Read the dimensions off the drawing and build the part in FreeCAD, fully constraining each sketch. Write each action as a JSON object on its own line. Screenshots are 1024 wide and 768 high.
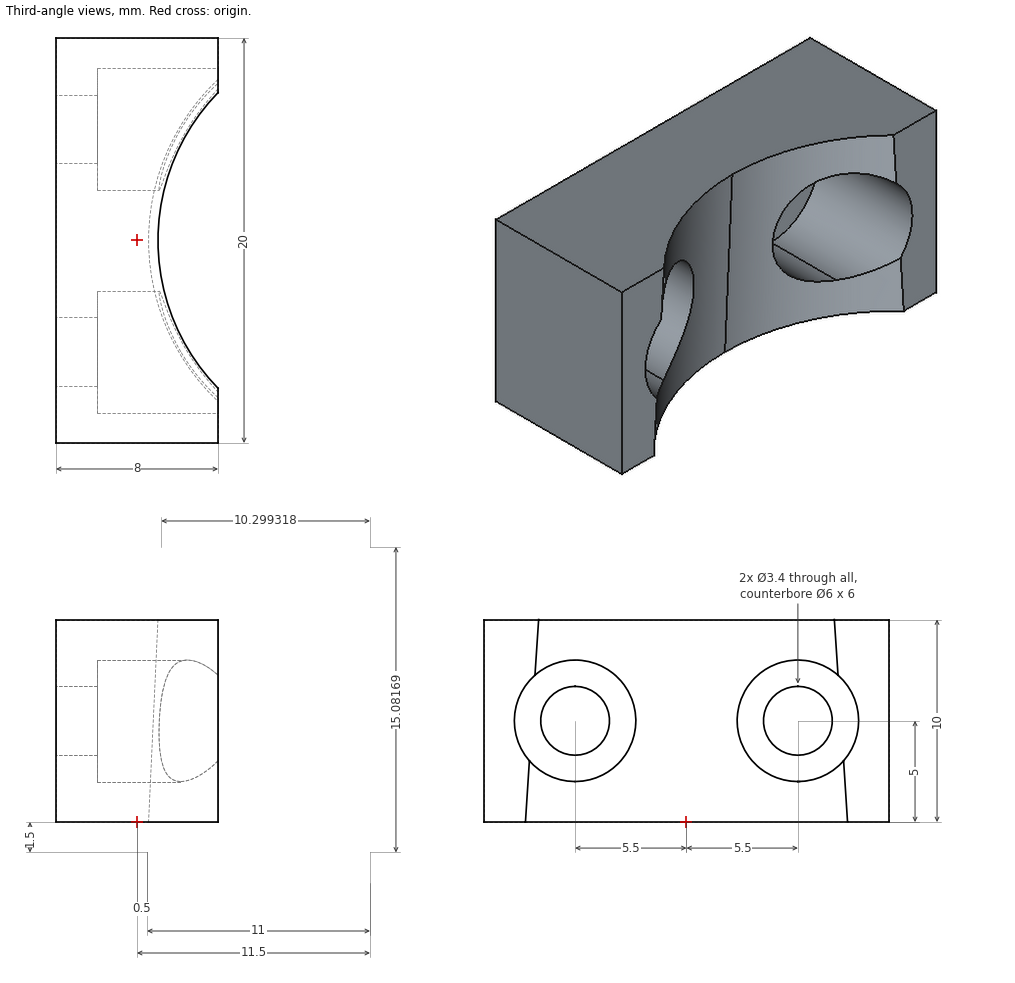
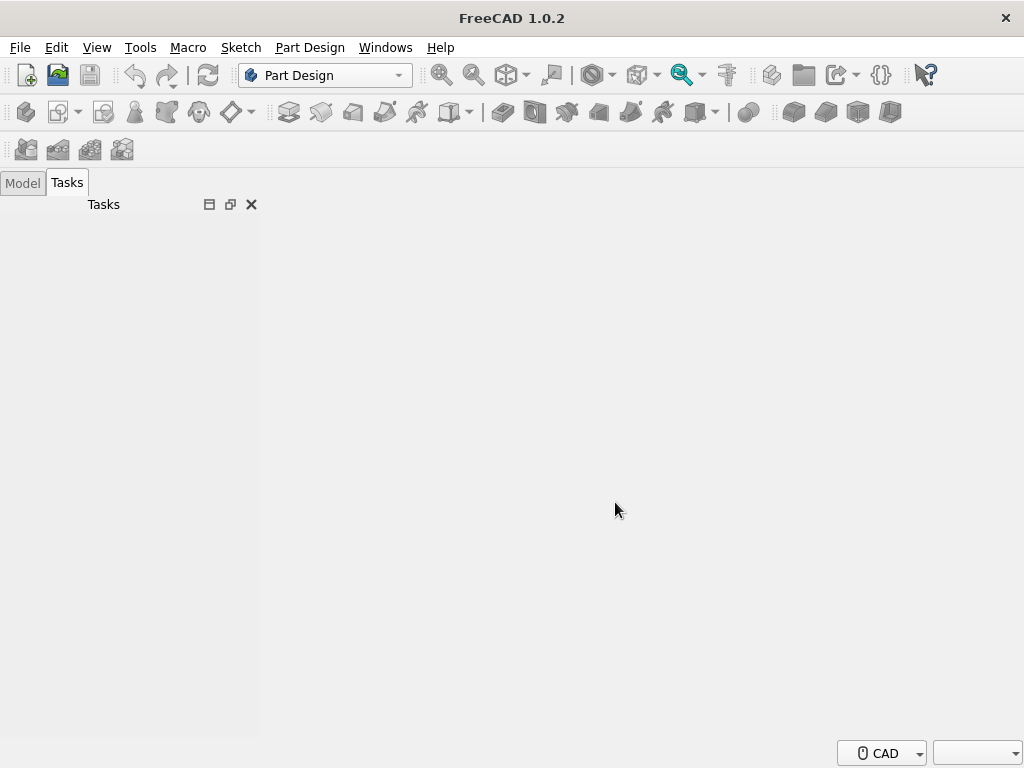
{"action": "key", "text": "ctrl+n"}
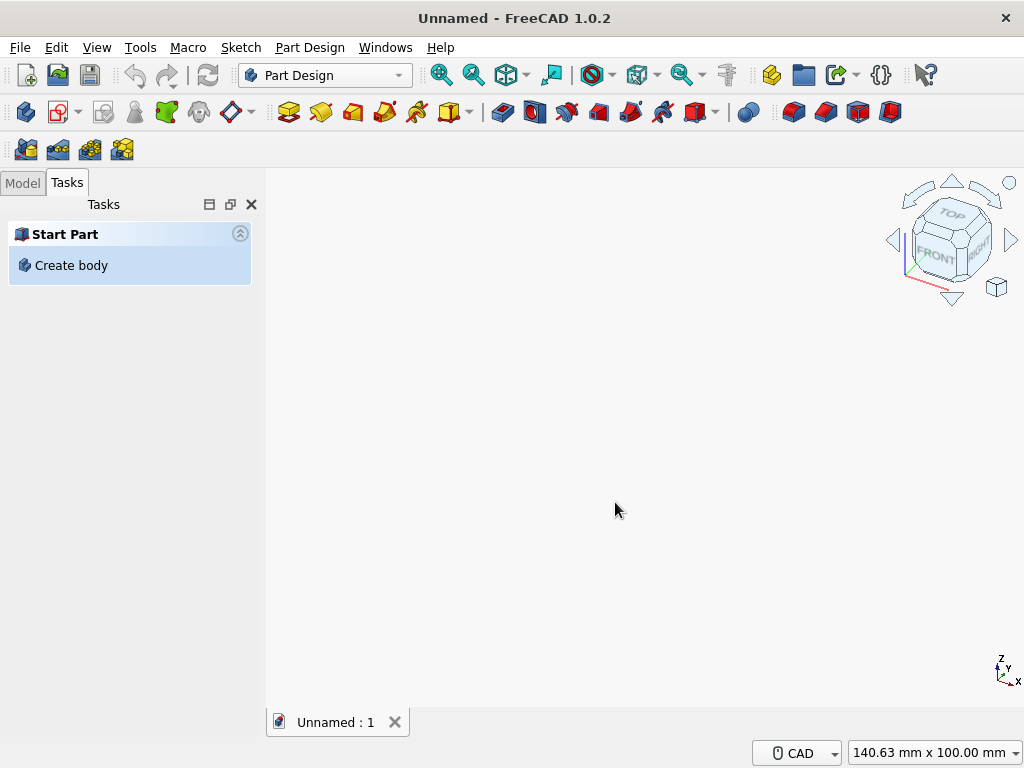
{"action": "left_click", "coordinate": [58, 112]}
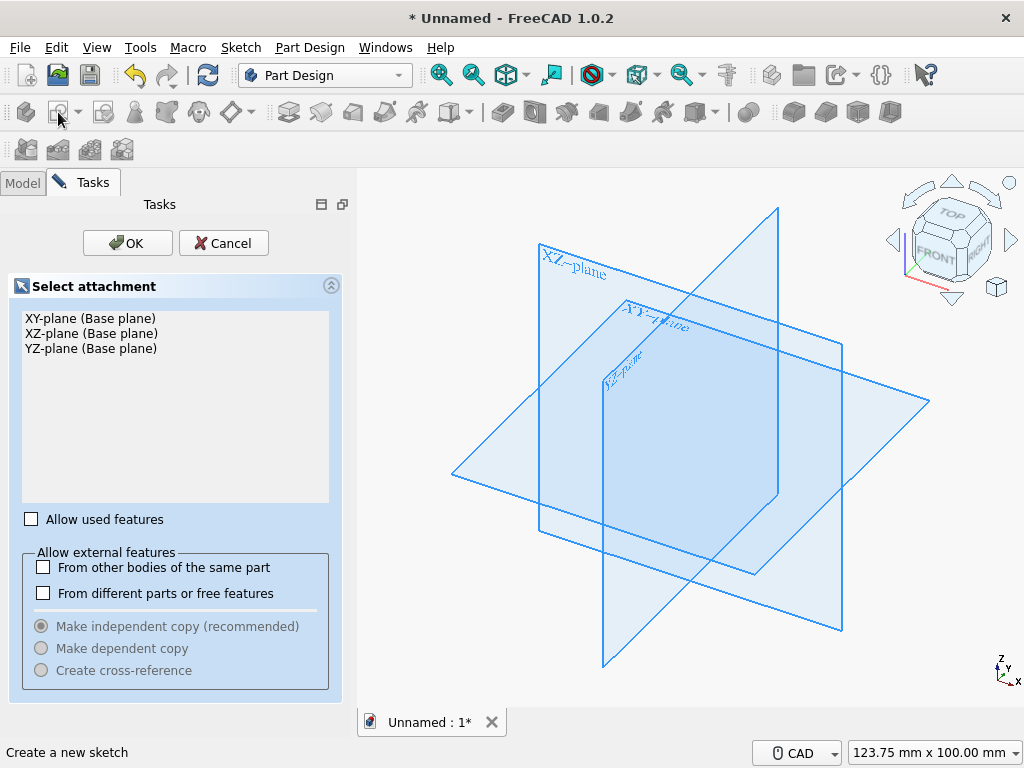
{"action": "left_click", "coordinate": [82, 318]}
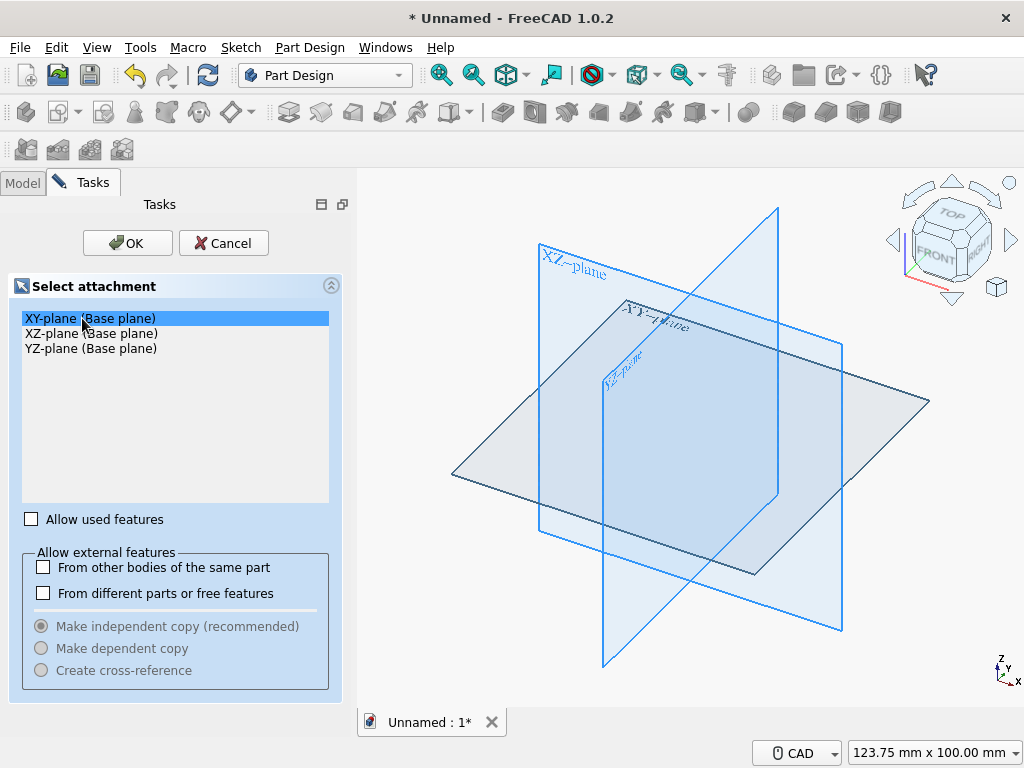
{"action": "left_click", "coordinate": [128, 243]}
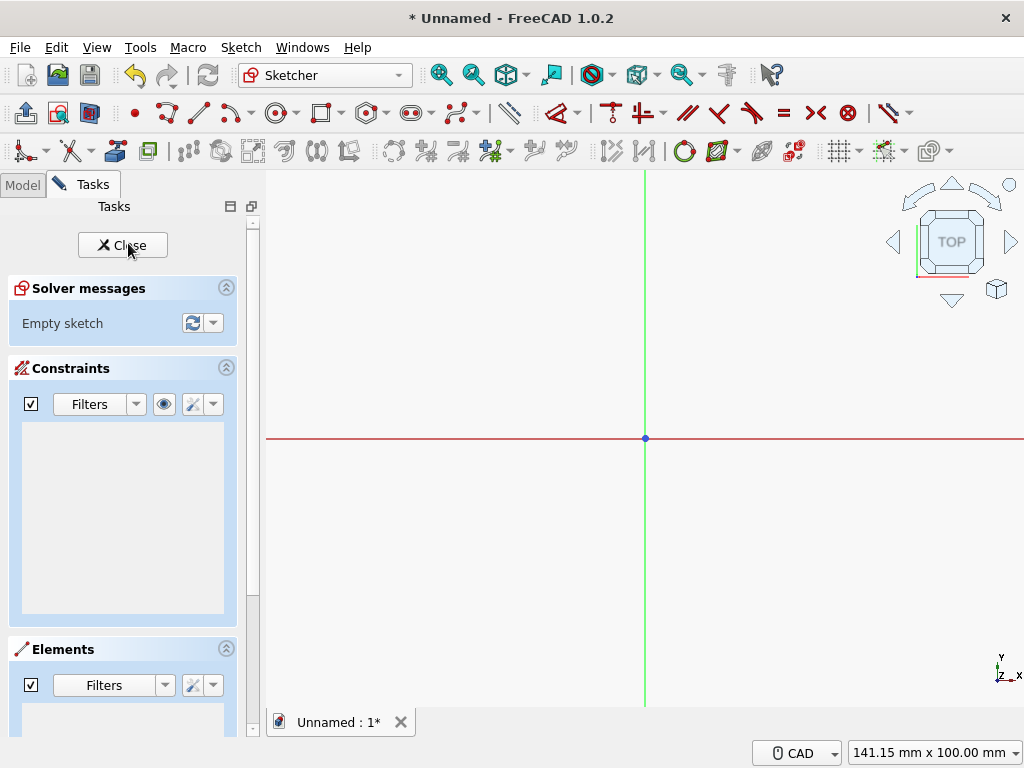
{"action": "scroll", "coordinate": [675, 438], "scroll_direction": "up", "scroll_amount": 6}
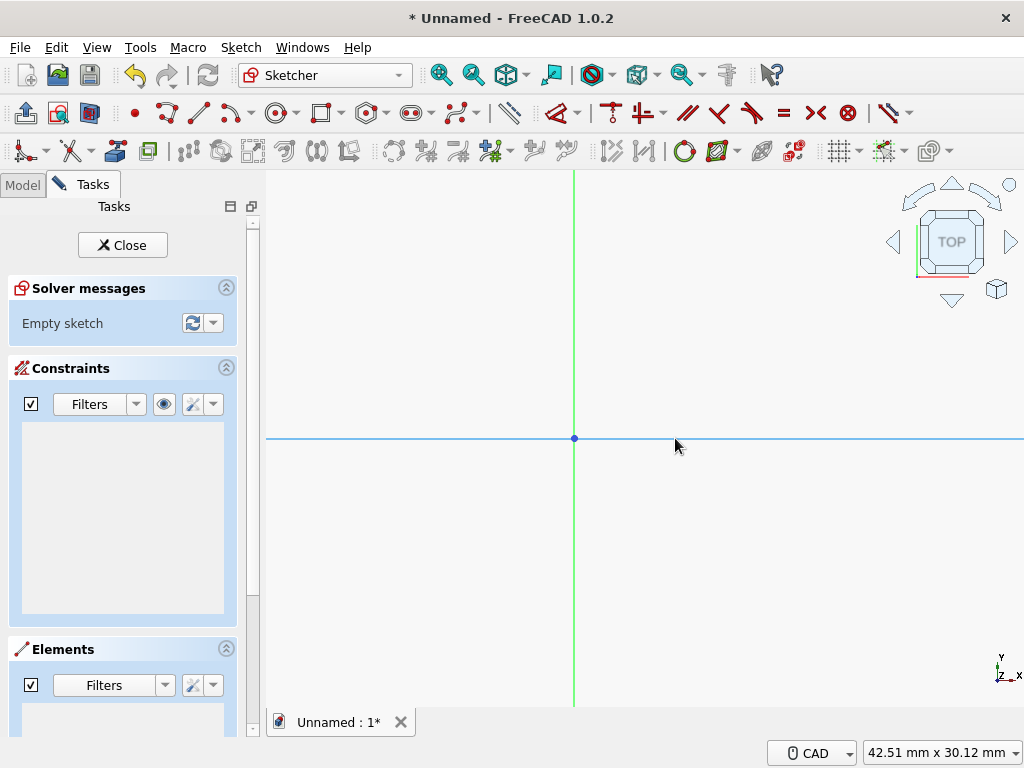
{"action": "key", "text": "g v"}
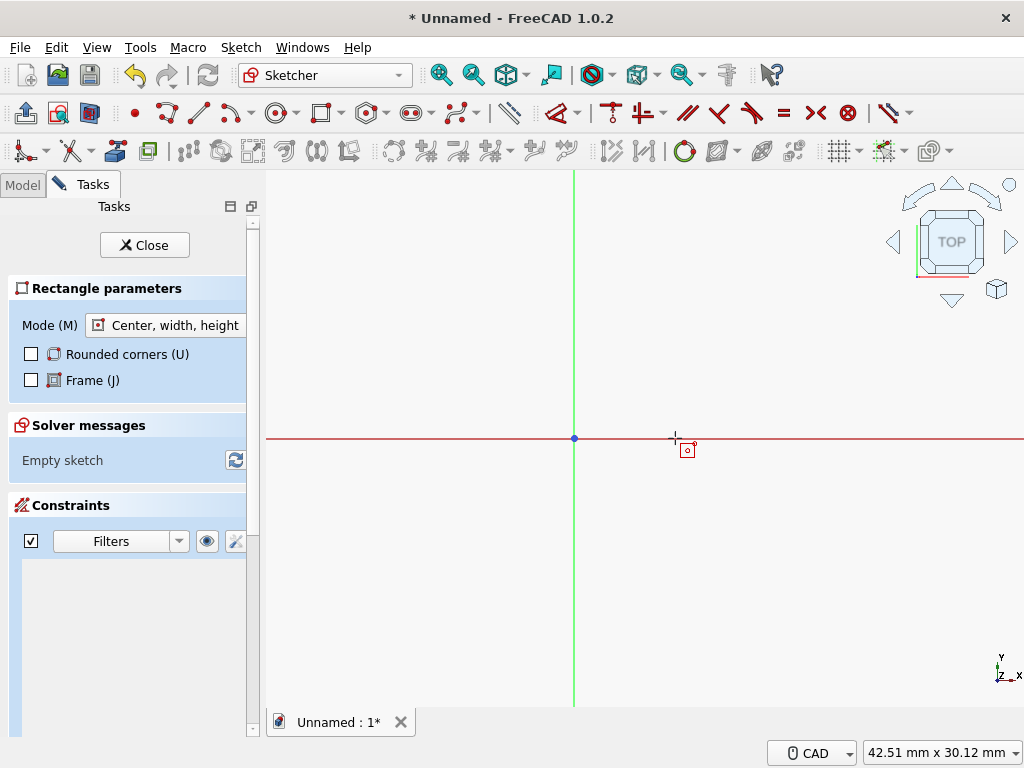
{"action": "left_click", "coordinate": [574, 438]}
{"action": "left_click", "coordinate": [645, 260]}
{"action": "key", "text": "Escape"}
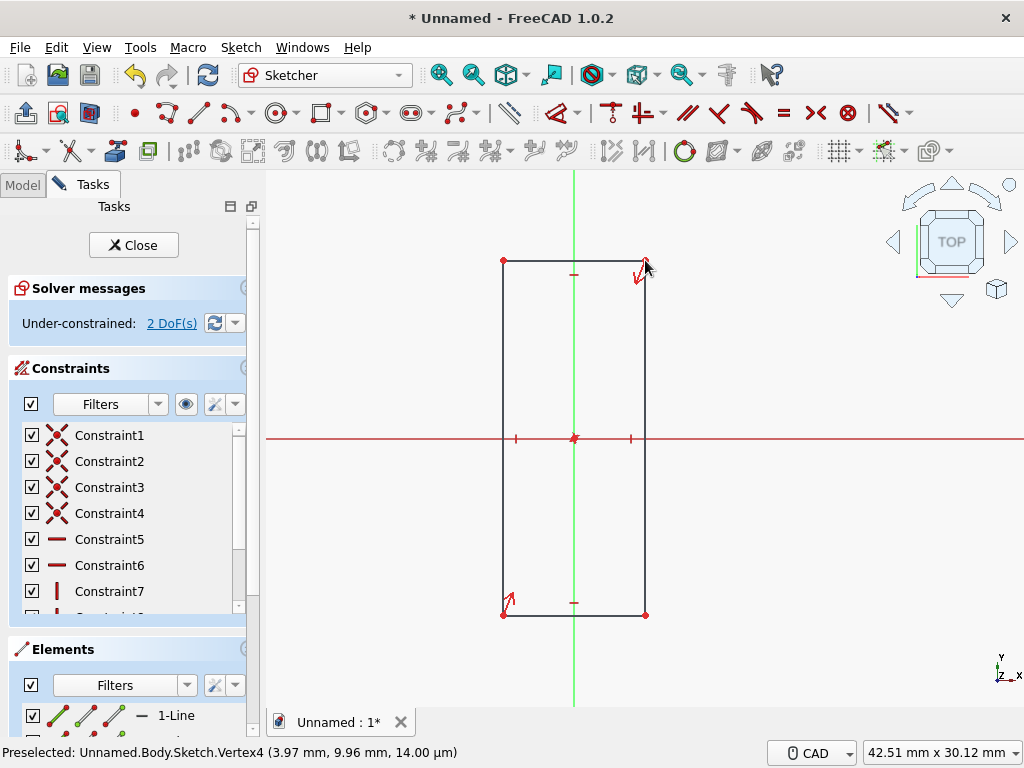
{"action": "key", "text": "d"}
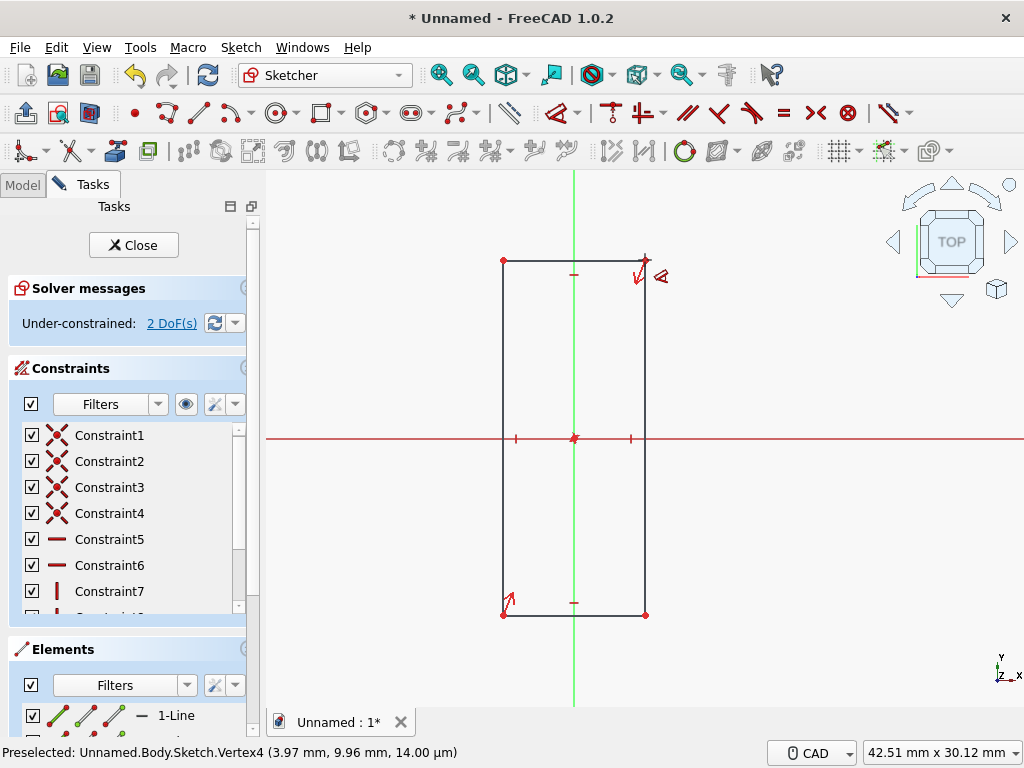
{"action": "left_click", "coordinate": [546, 616]}
{"action": "left_click", "coordinate": [542, 650]}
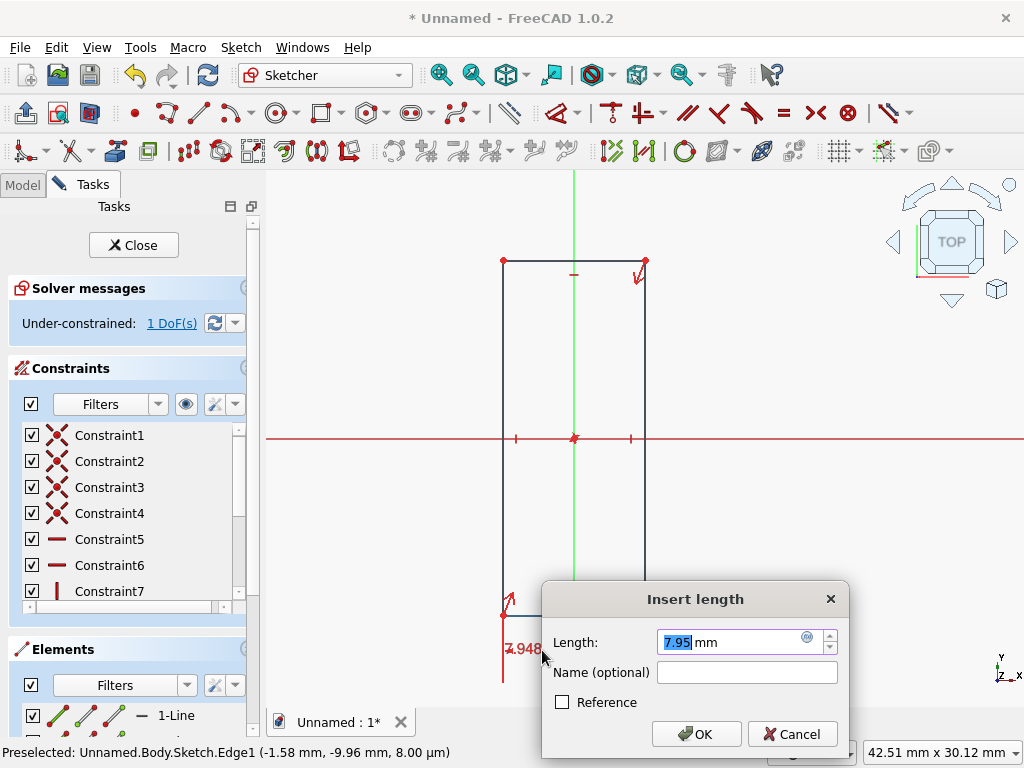
{"action": "type", "text": "8"}
{"action": "key", "text": "Return"}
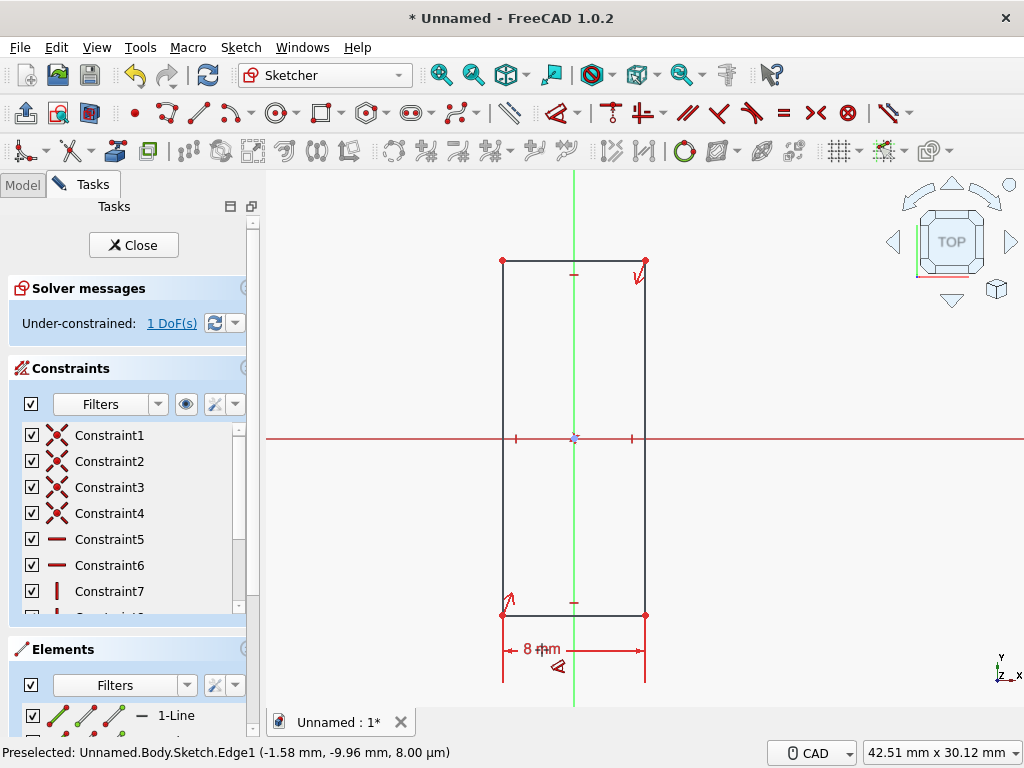
{"action": "left_click", "coordinate": [645, 510]}
{"action": "left_click", "coordinate": [679, 357]}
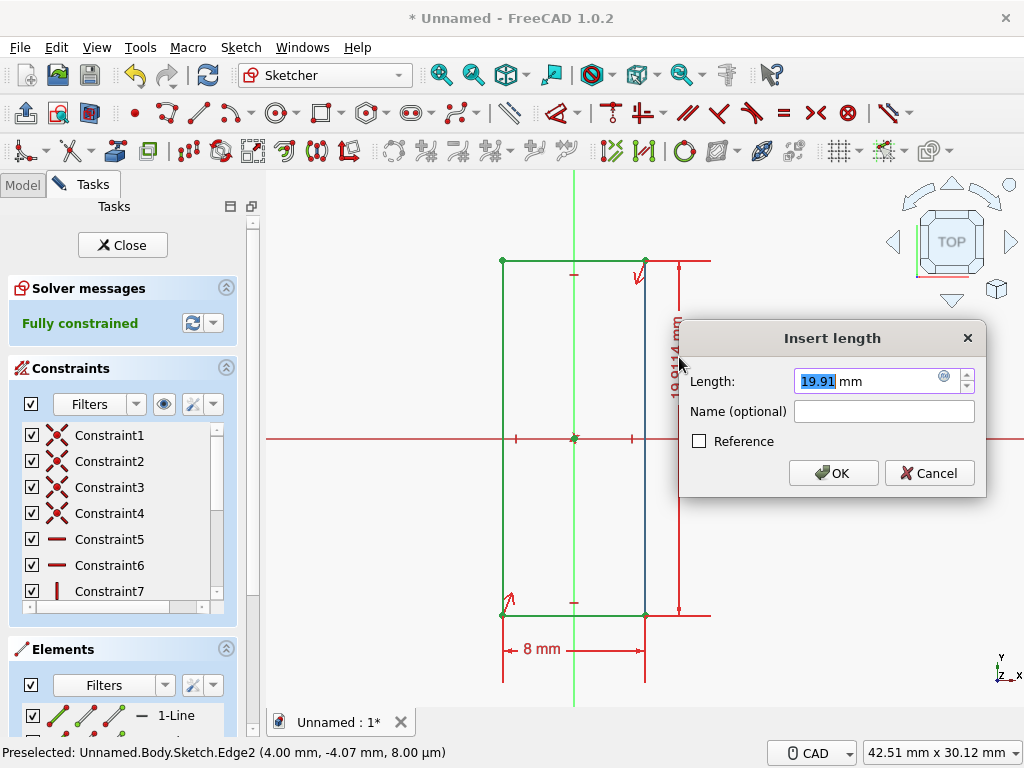
{"action": "type", "text": "20"}
{"action": "key", "text": "Return"}
{"action": "key", "text": "Escape"}